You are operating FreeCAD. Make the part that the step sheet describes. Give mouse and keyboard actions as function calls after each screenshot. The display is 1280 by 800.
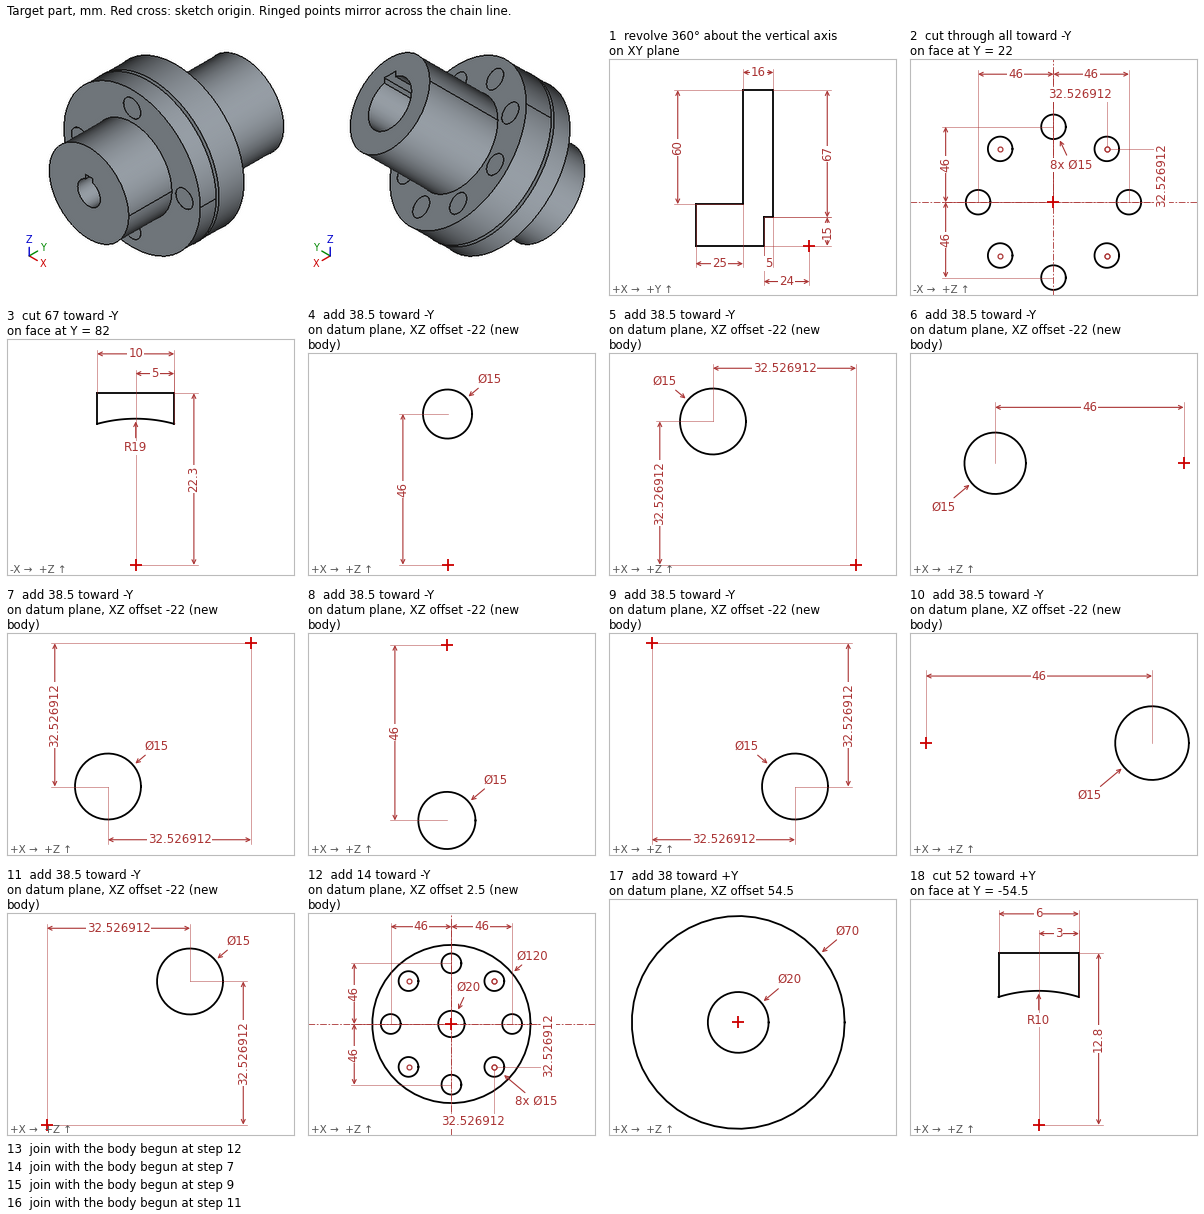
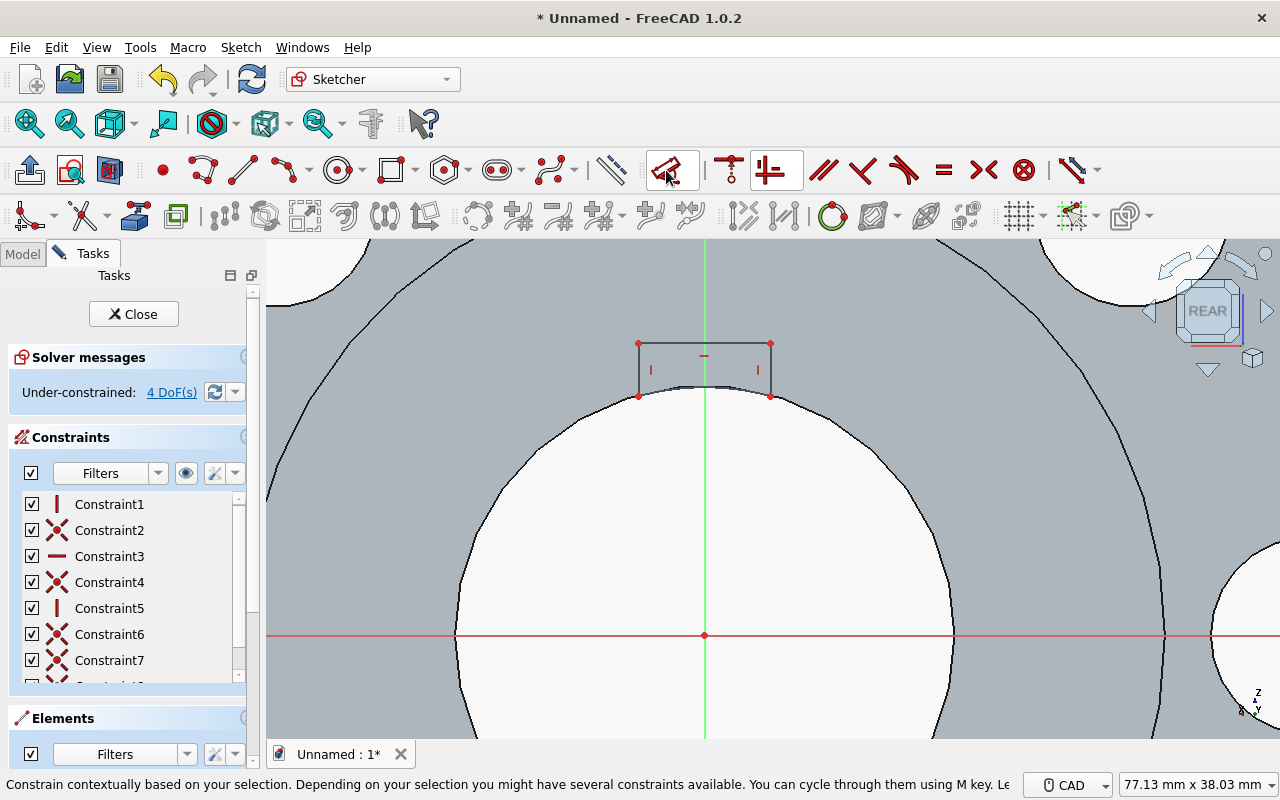
click(731, 389)
click(734, 357)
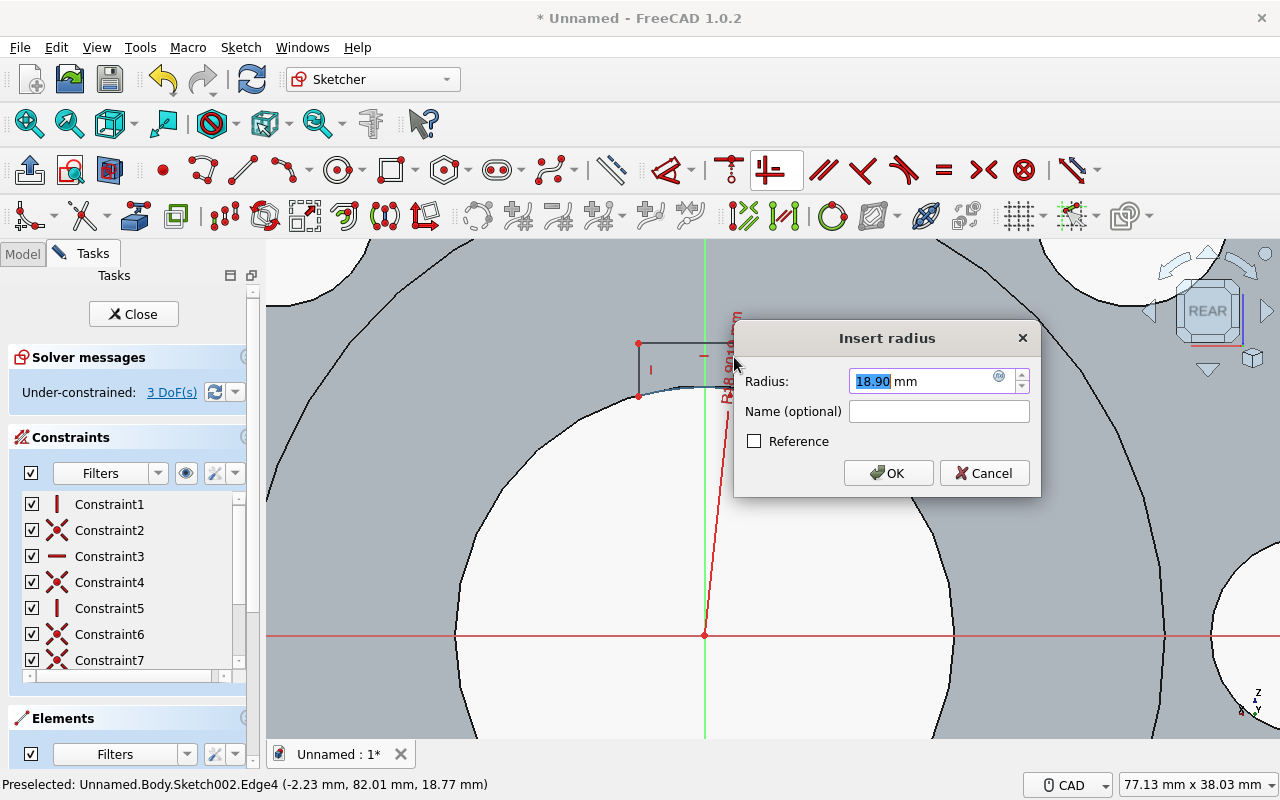
text(19)
key(Return)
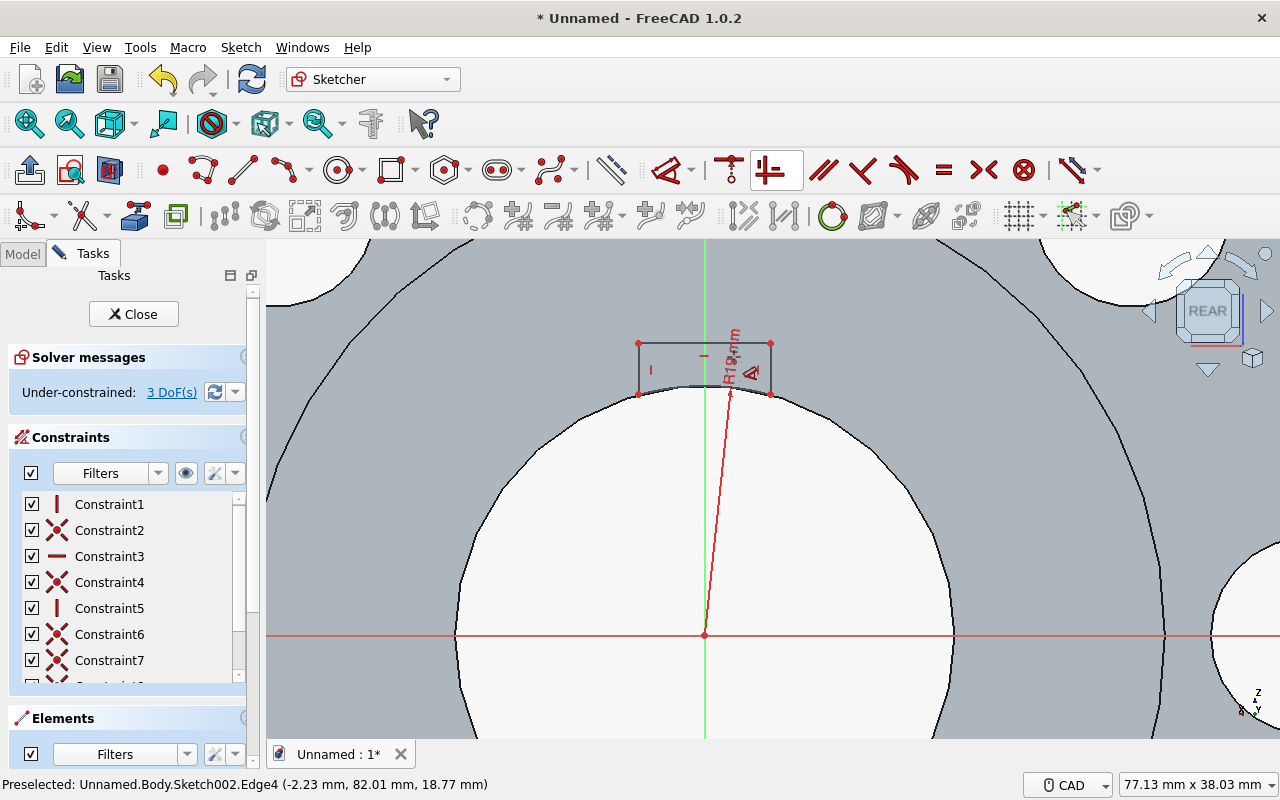
click(731, 343)
click(674, 309)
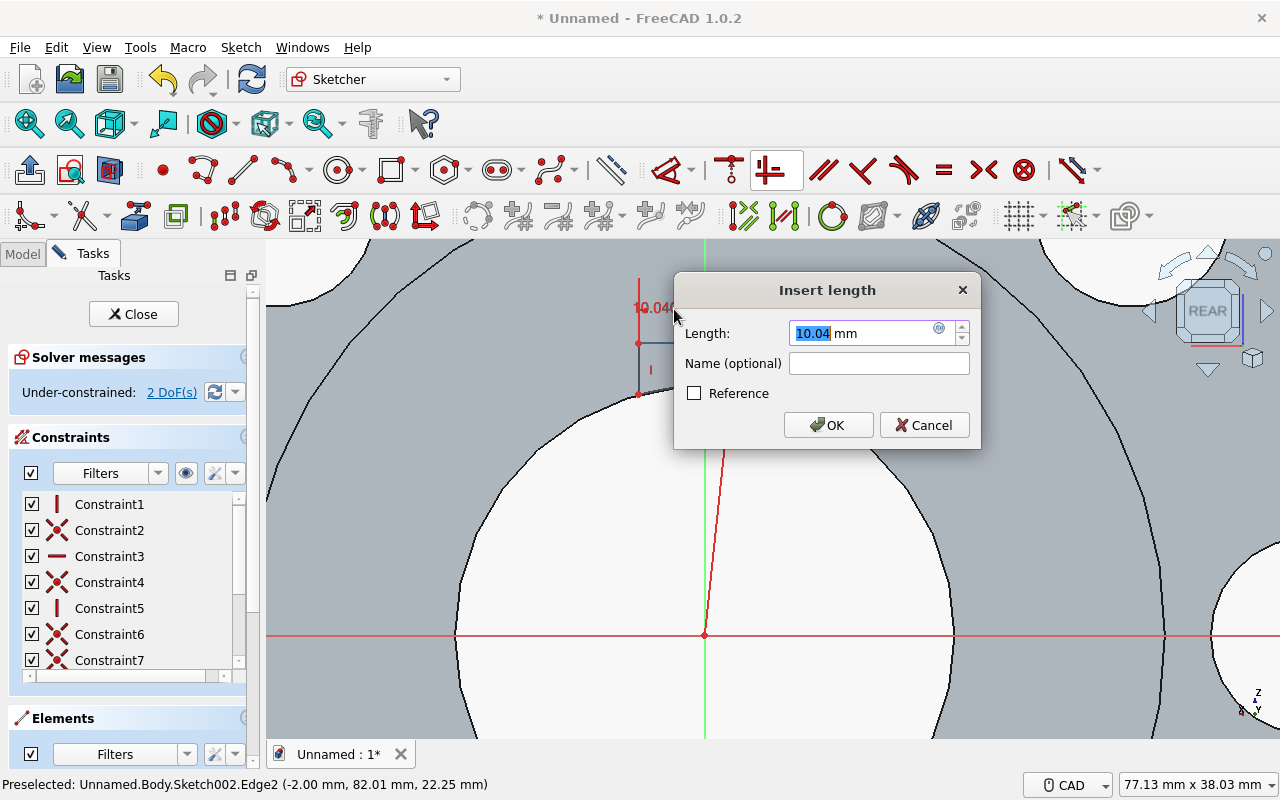
text(10)
key(Return)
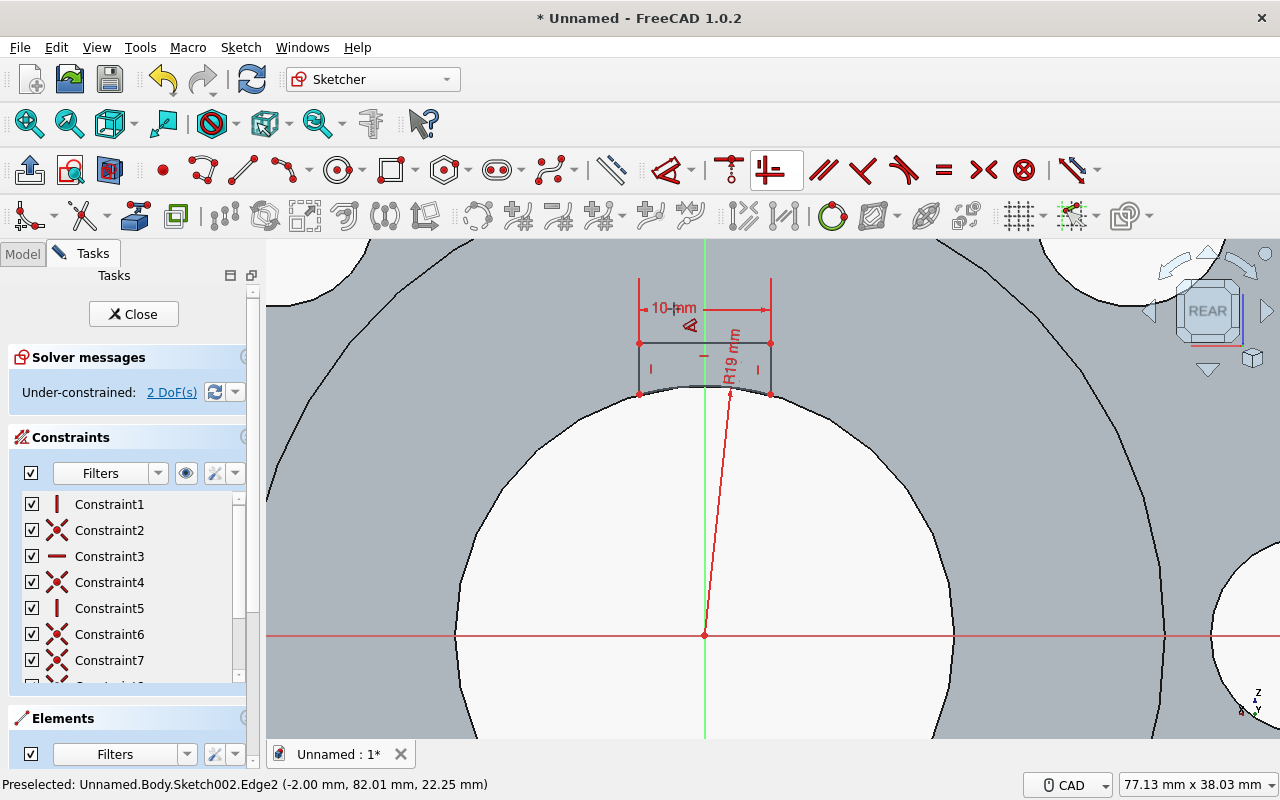
click(771, 395)
click(738, 670)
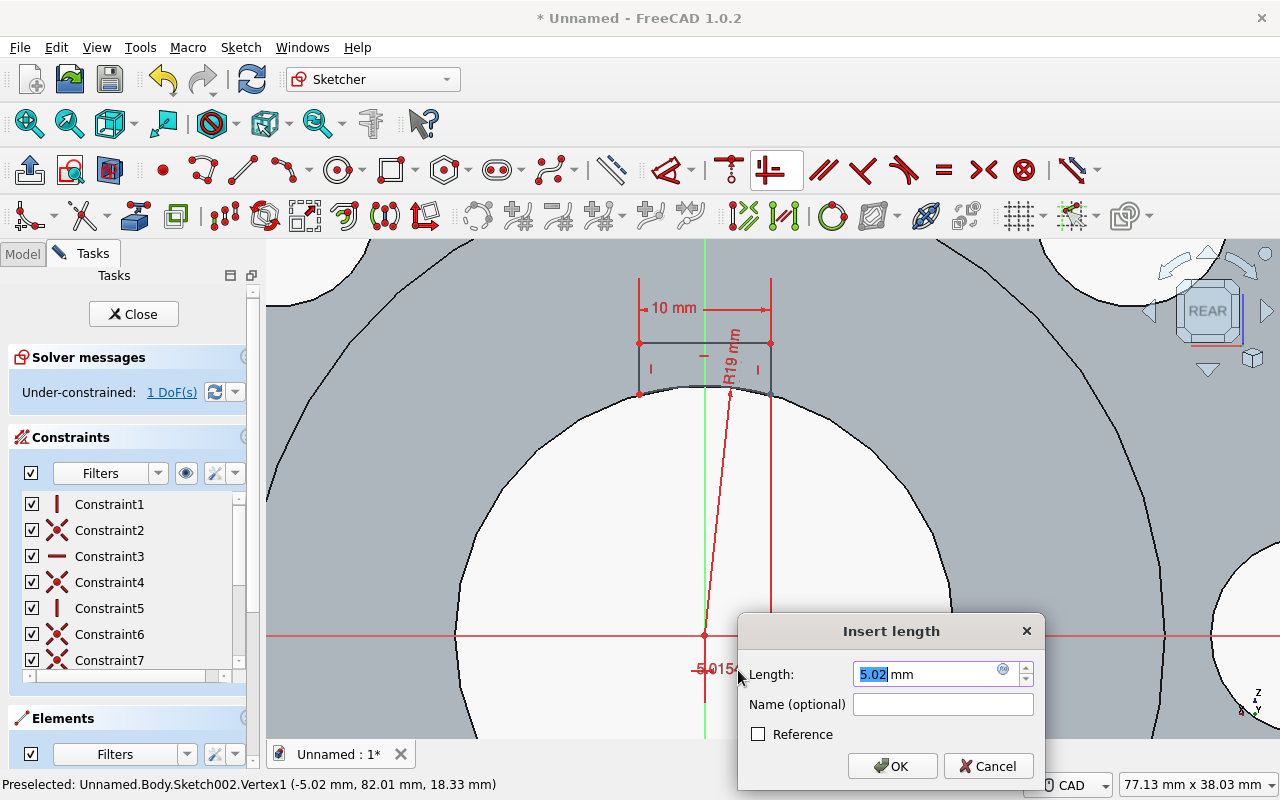
text(5)
key(Return)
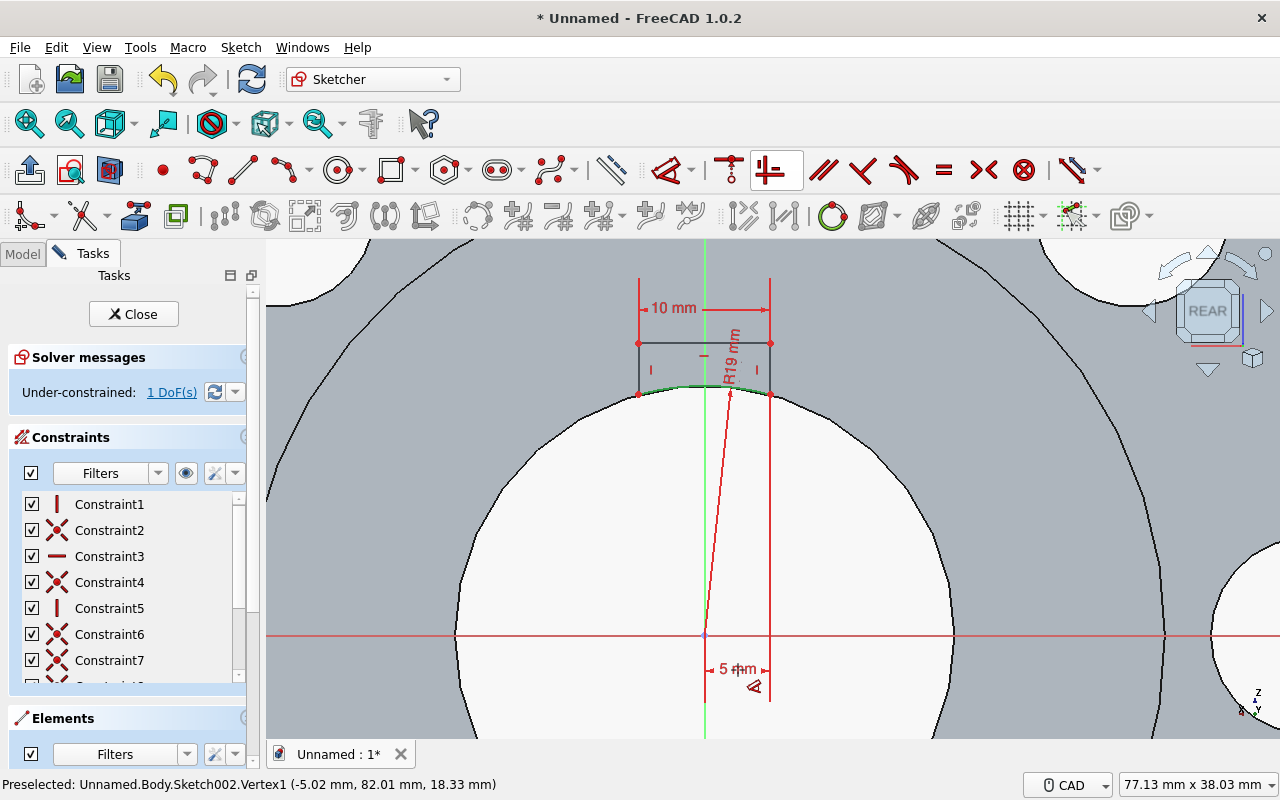
click(770, 343)
click(804, 489)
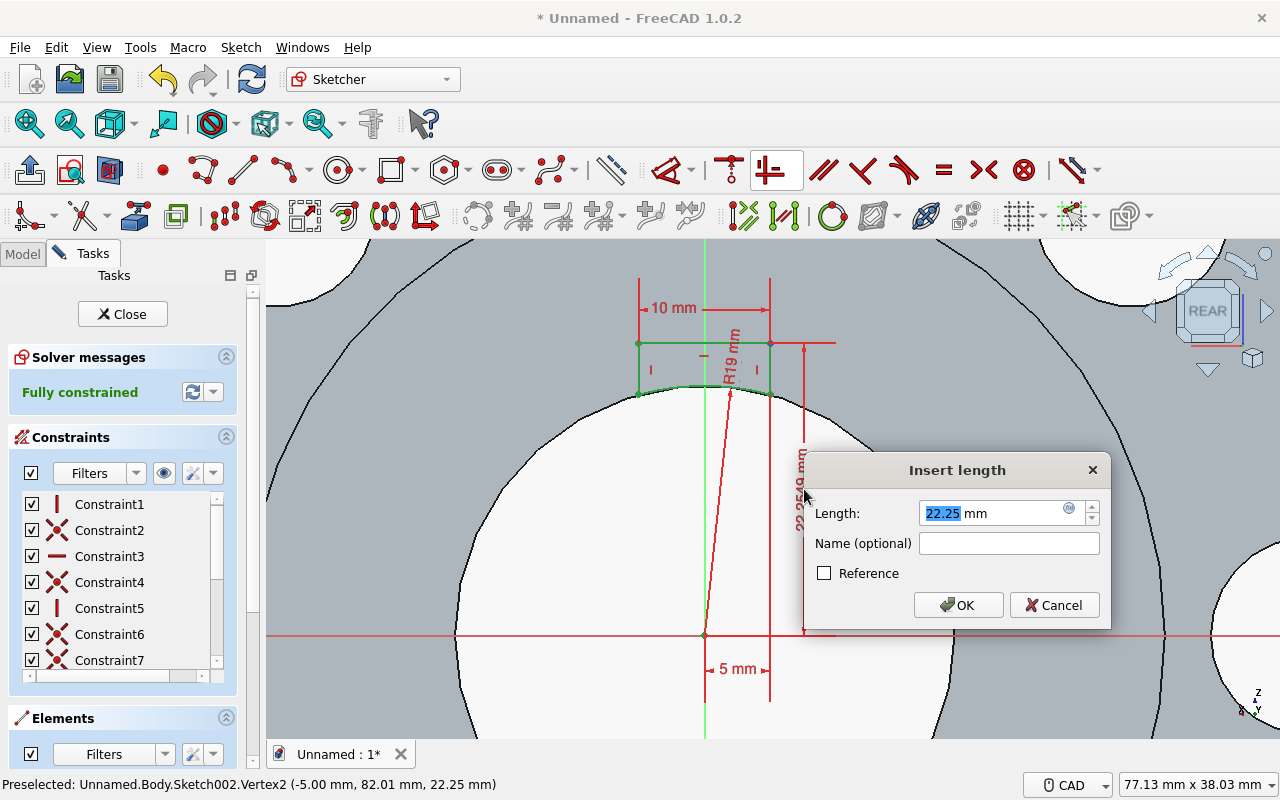
text(22.3)
key(Return)
key(Escape)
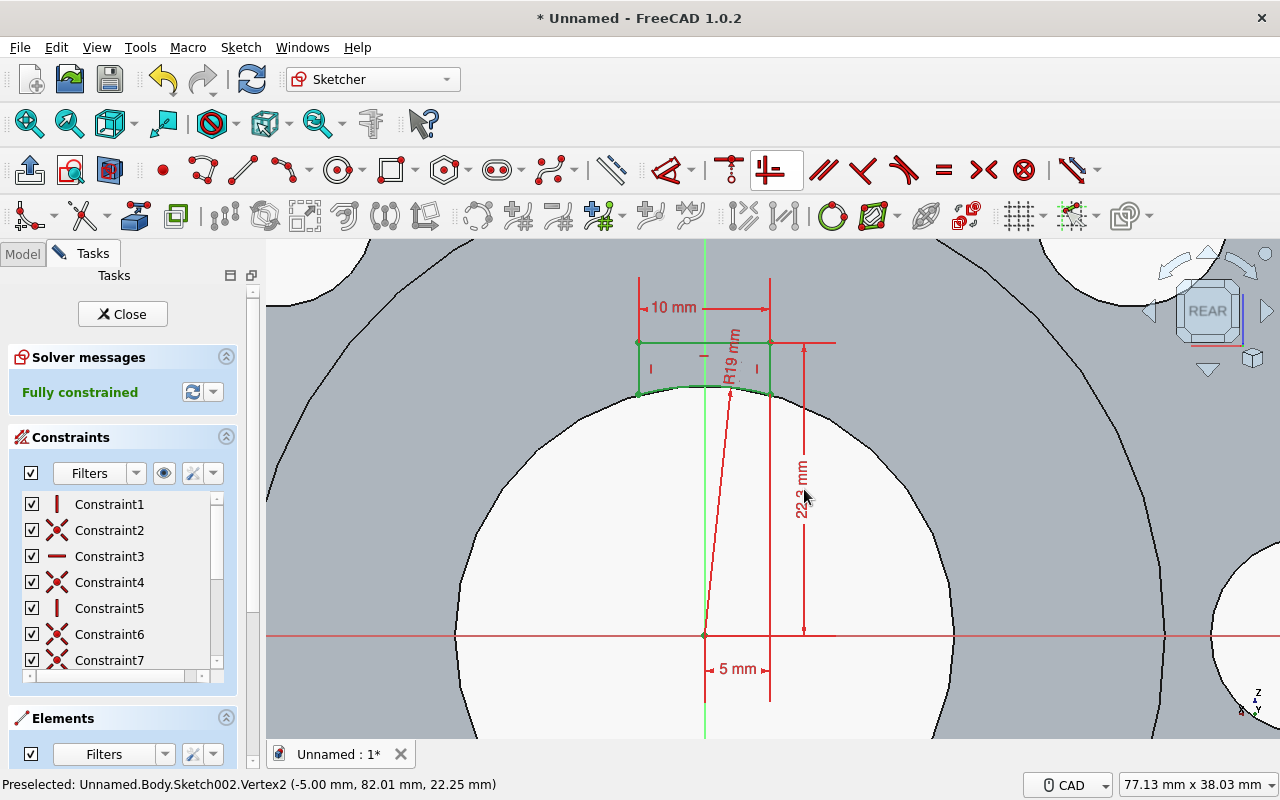
click(123, 314)